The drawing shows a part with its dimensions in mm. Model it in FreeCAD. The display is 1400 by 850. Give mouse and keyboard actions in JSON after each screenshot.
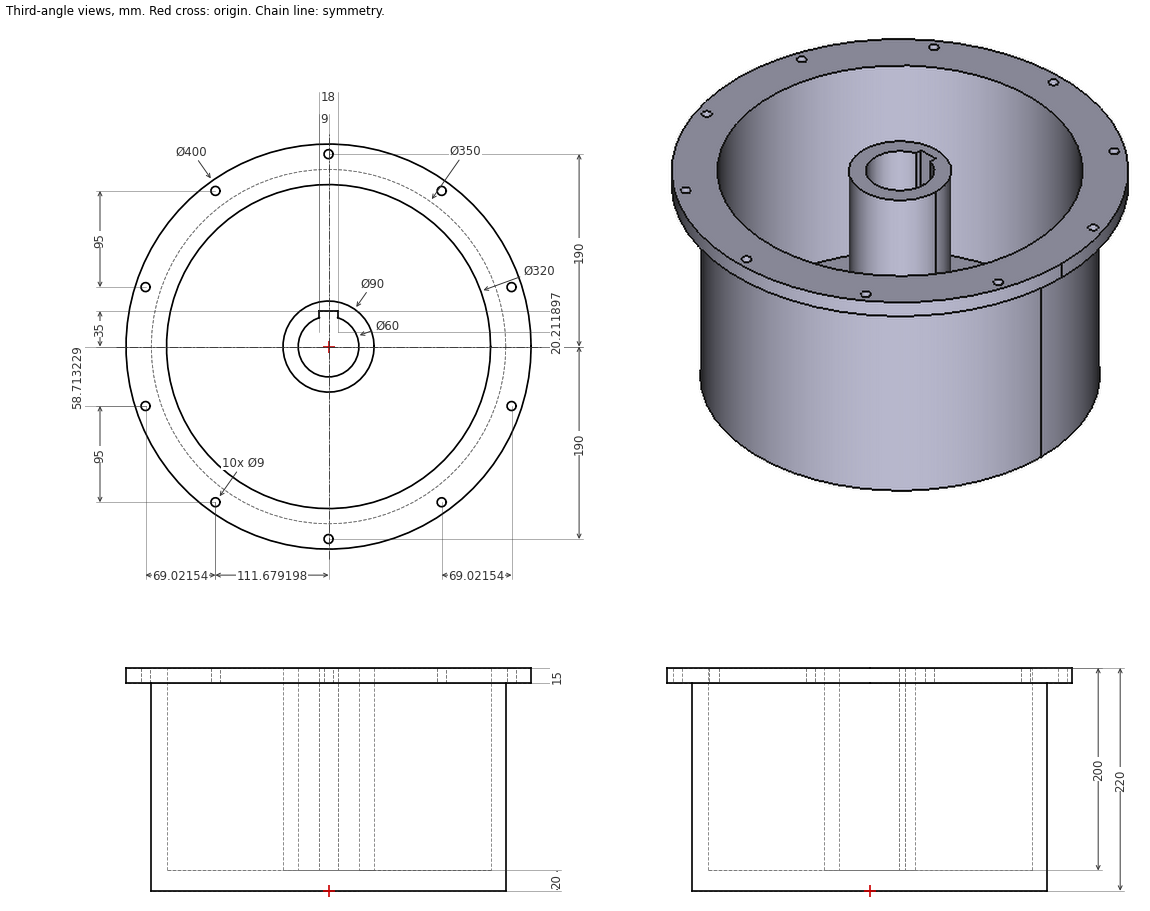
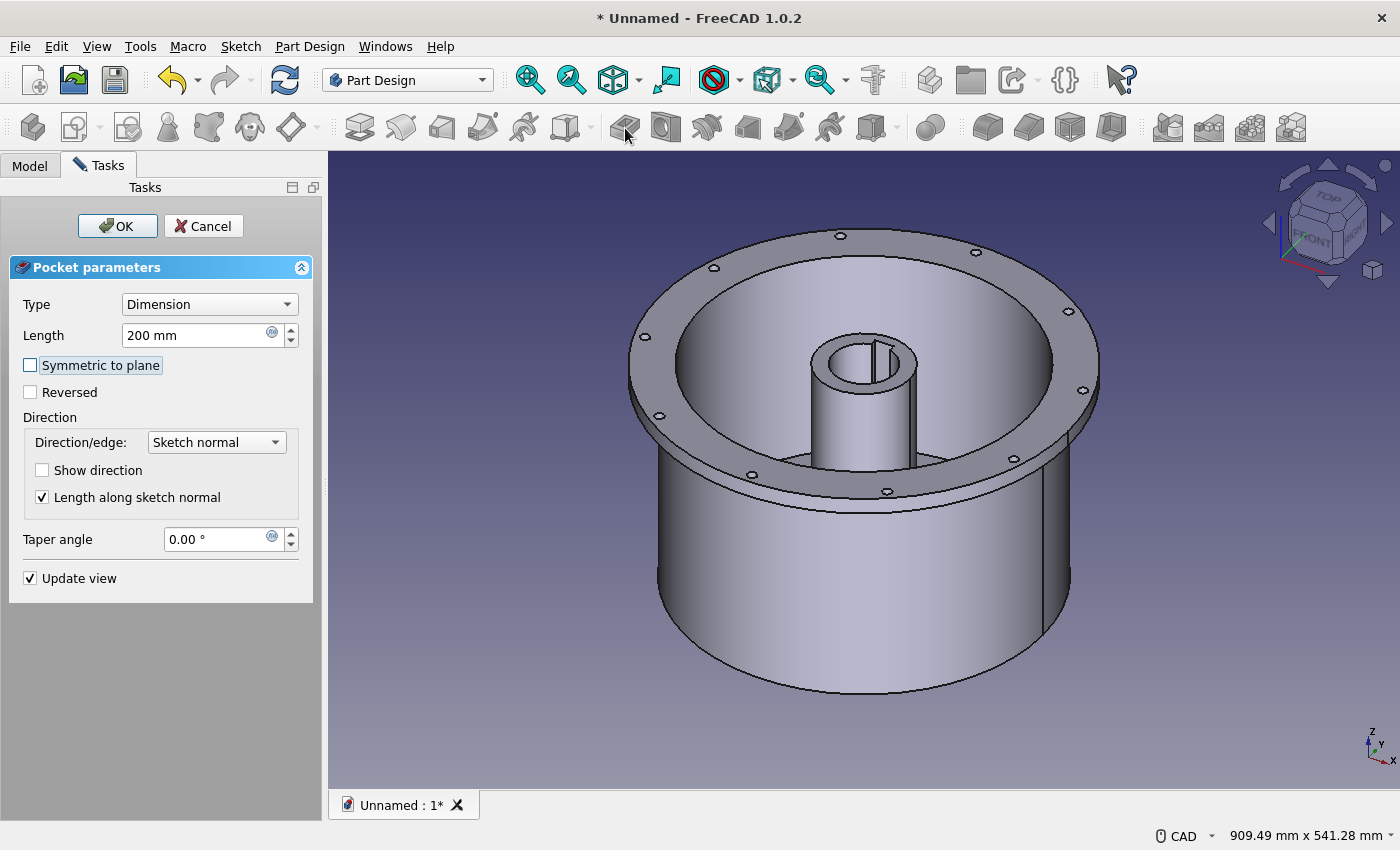
{"action": "left_click", "coordinate": [118, 226]}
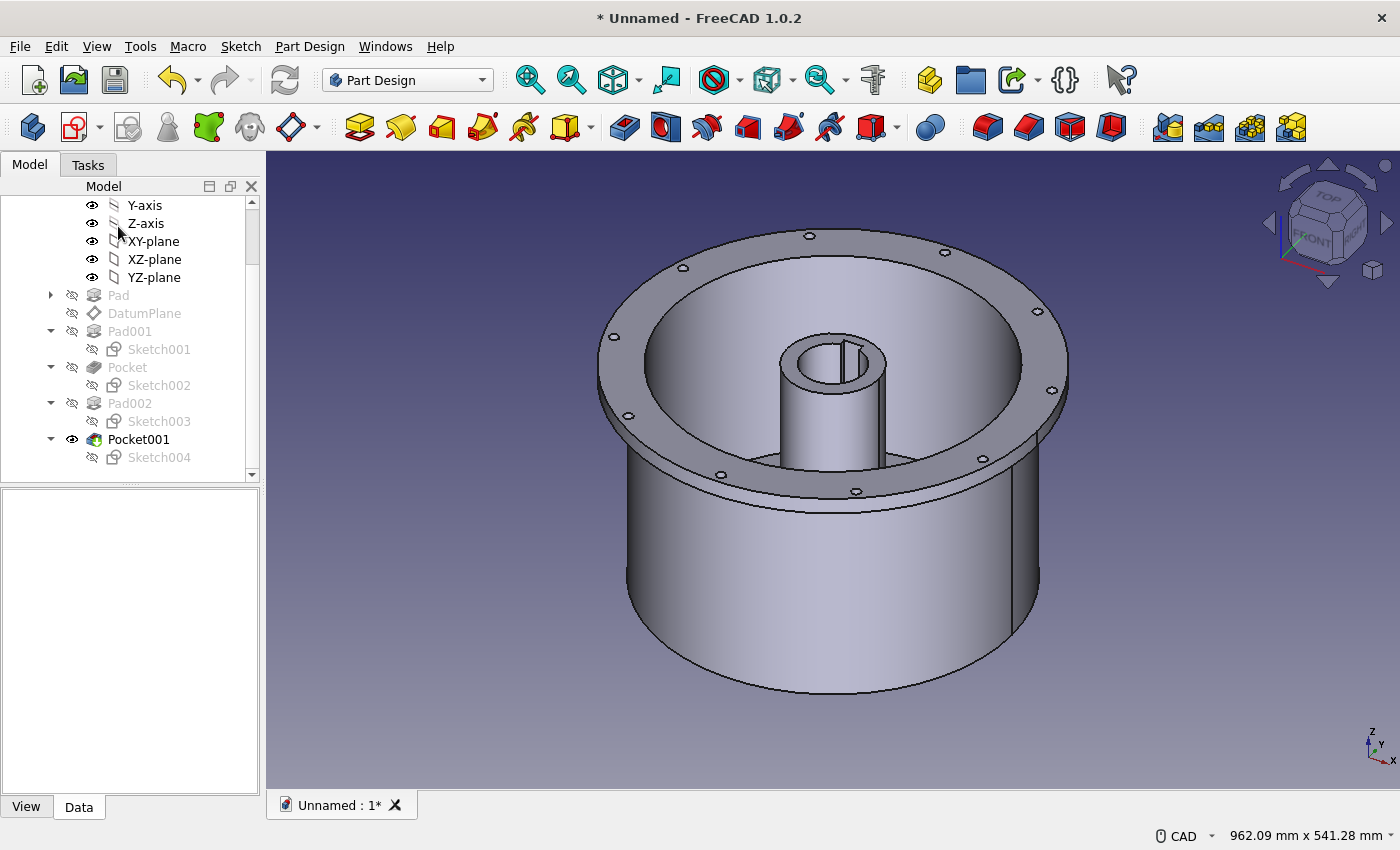
{"action": "key", "text": "0"}